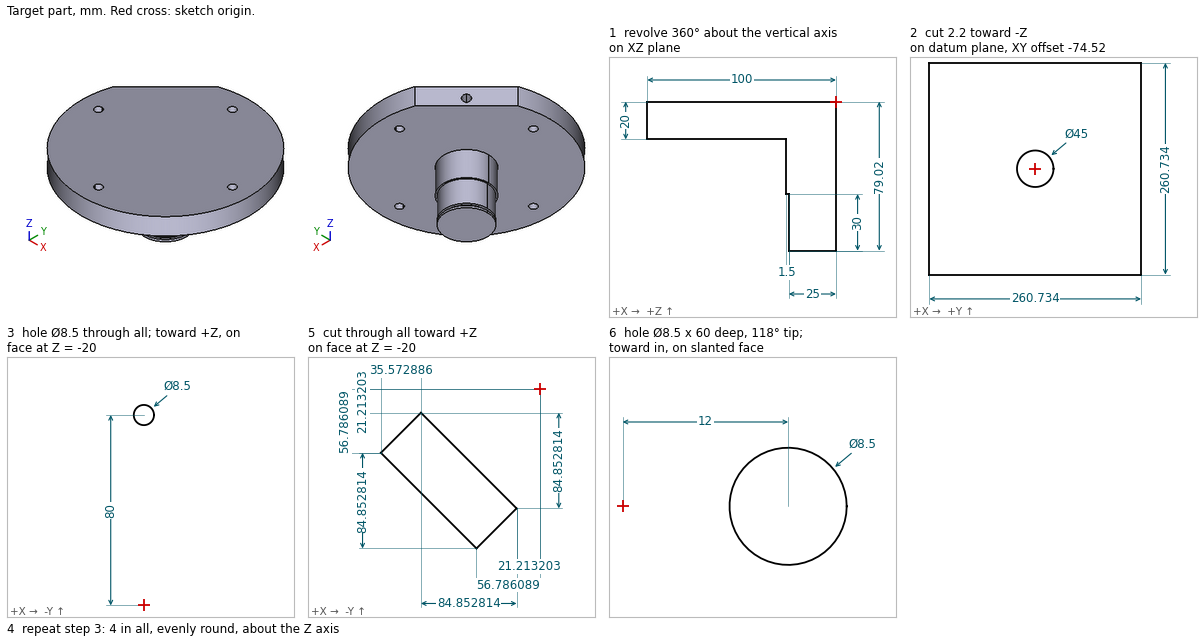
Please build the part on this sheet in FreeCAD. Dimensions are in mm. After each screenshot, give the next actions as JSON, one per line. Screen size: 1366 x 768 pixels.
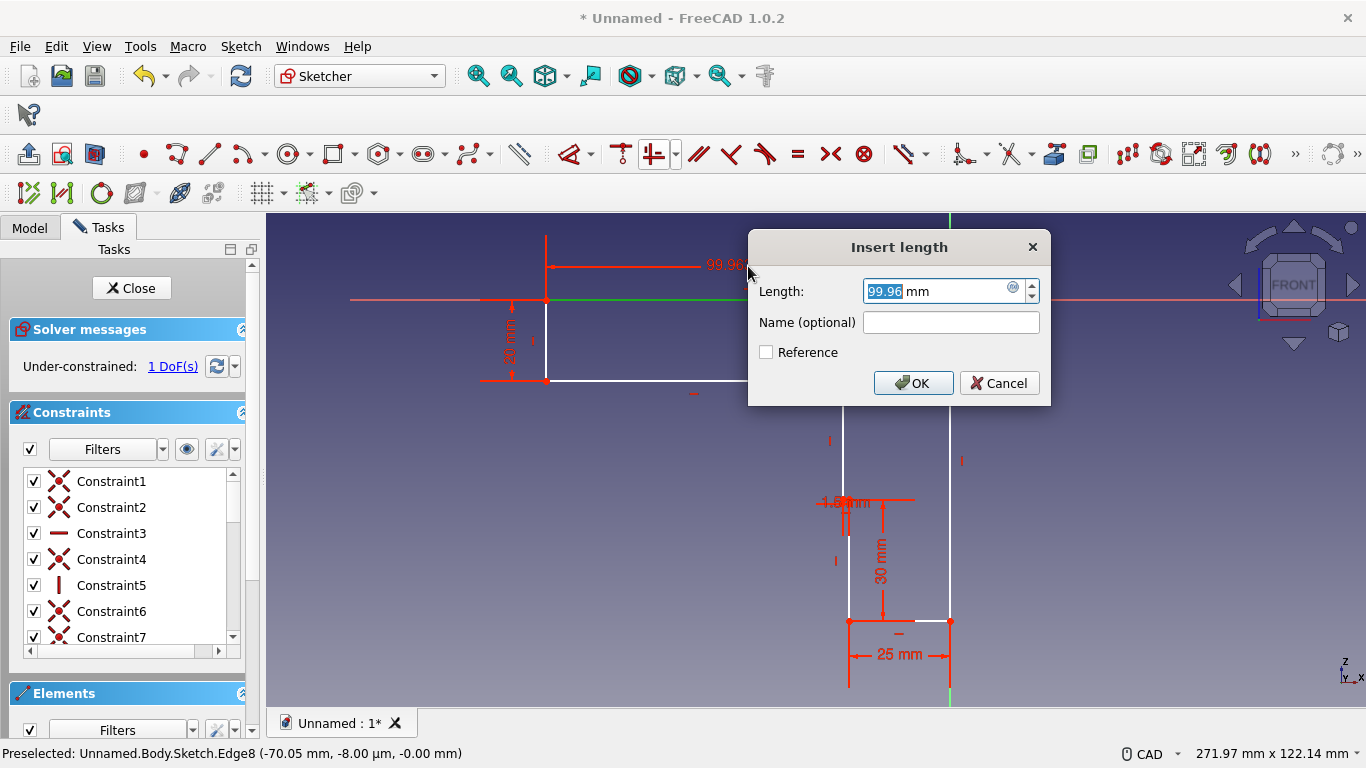
{"action": "type", "text": "100"}
{"action": "key", "text": "Return"}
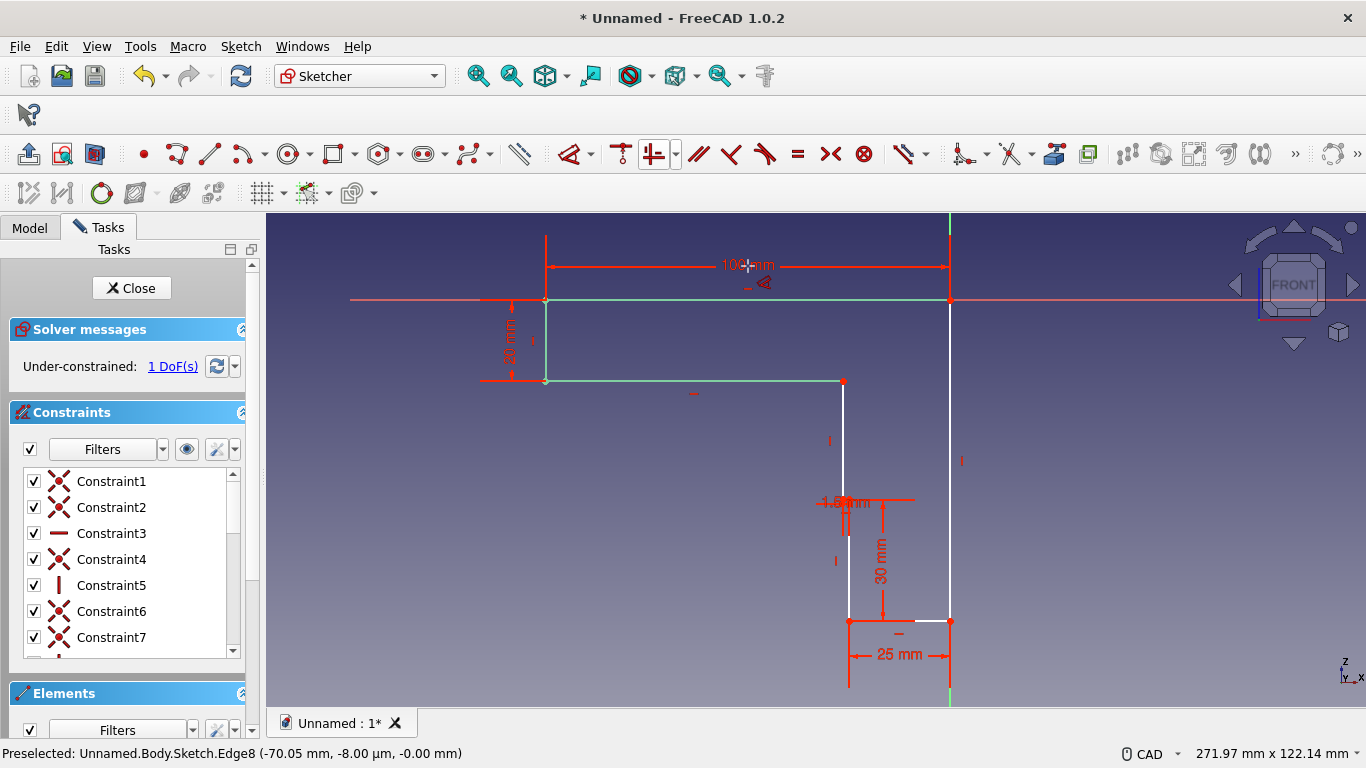
{"action": "left_click", "coordinate": [950, 397]}
{"action": "left_click", "coordinate": [984, 461]}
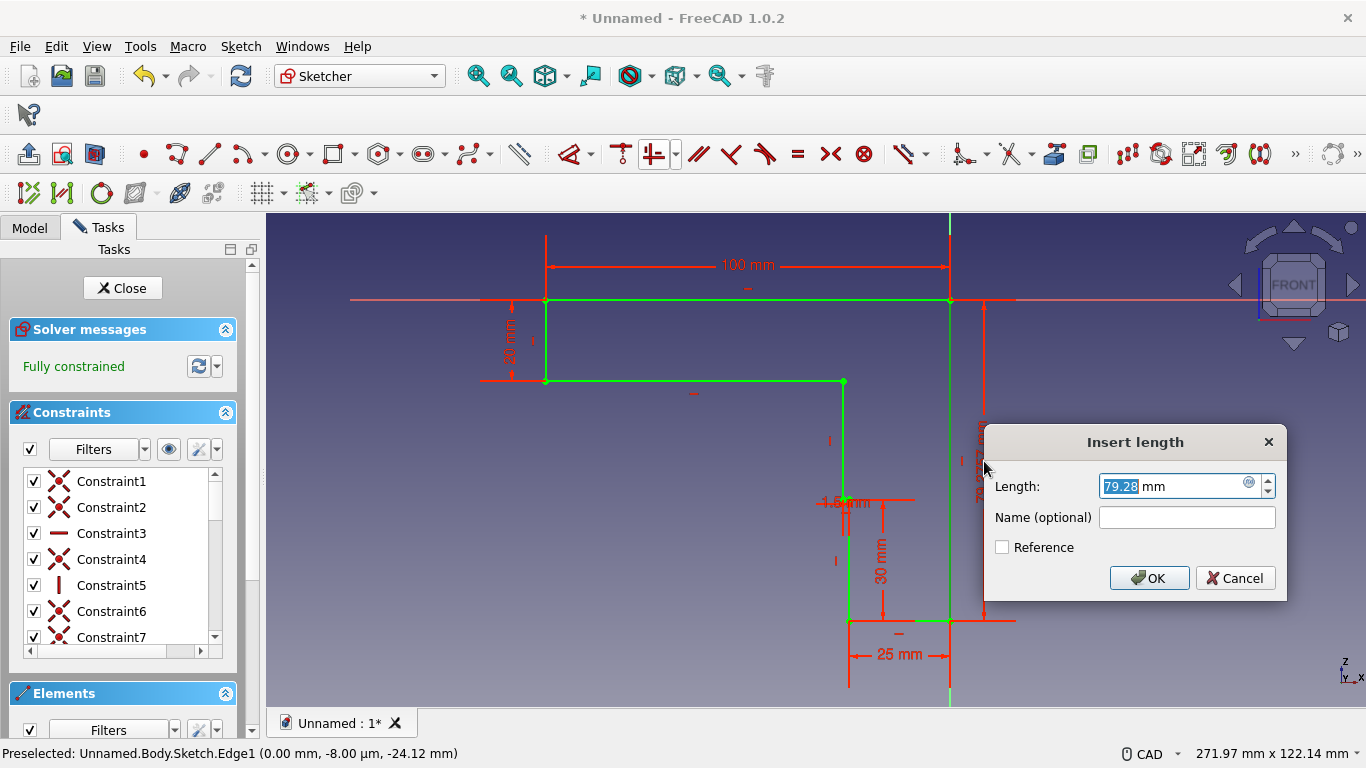
{"action": "type", "text": "79.02"}
{"action": "key", "text": "Return"}
{"action": "key", "text": "Escape"}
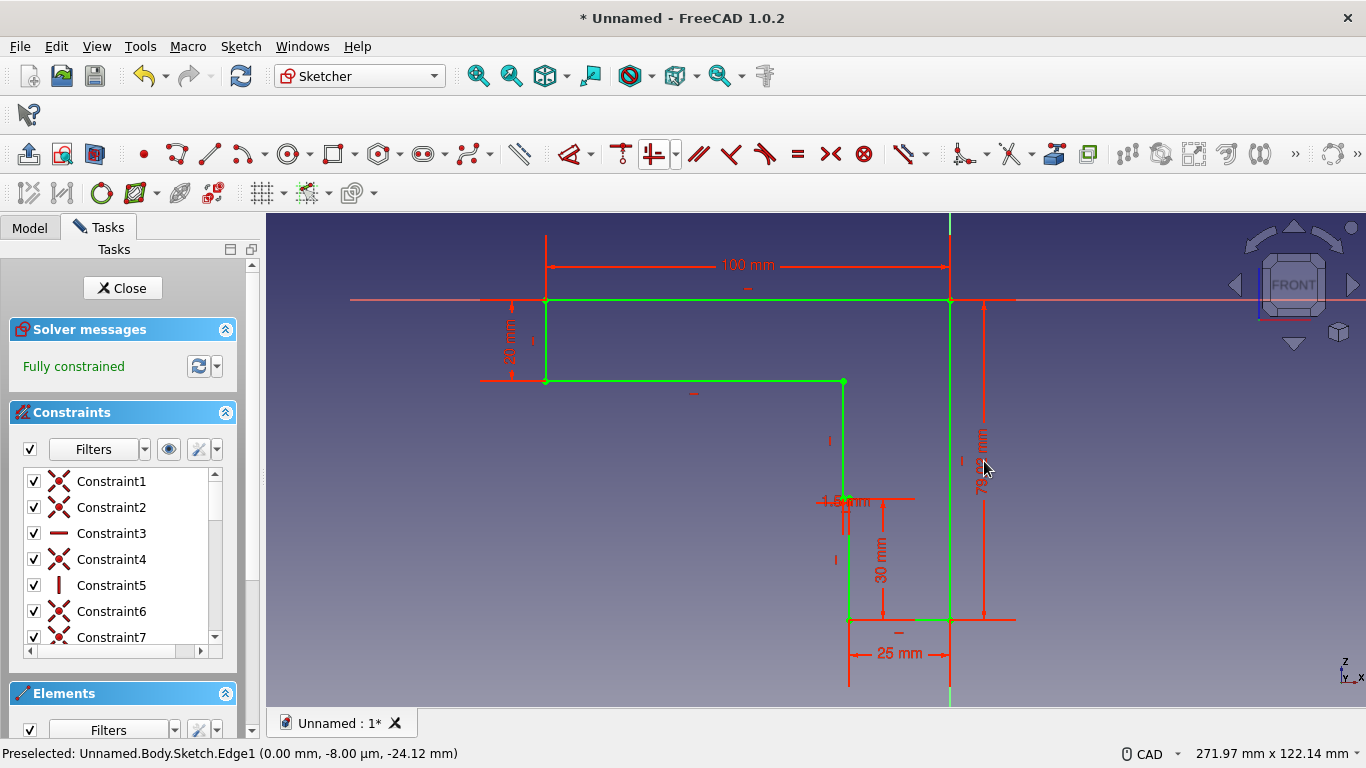
{"action": "left_click", "coordinate": [123, 288]}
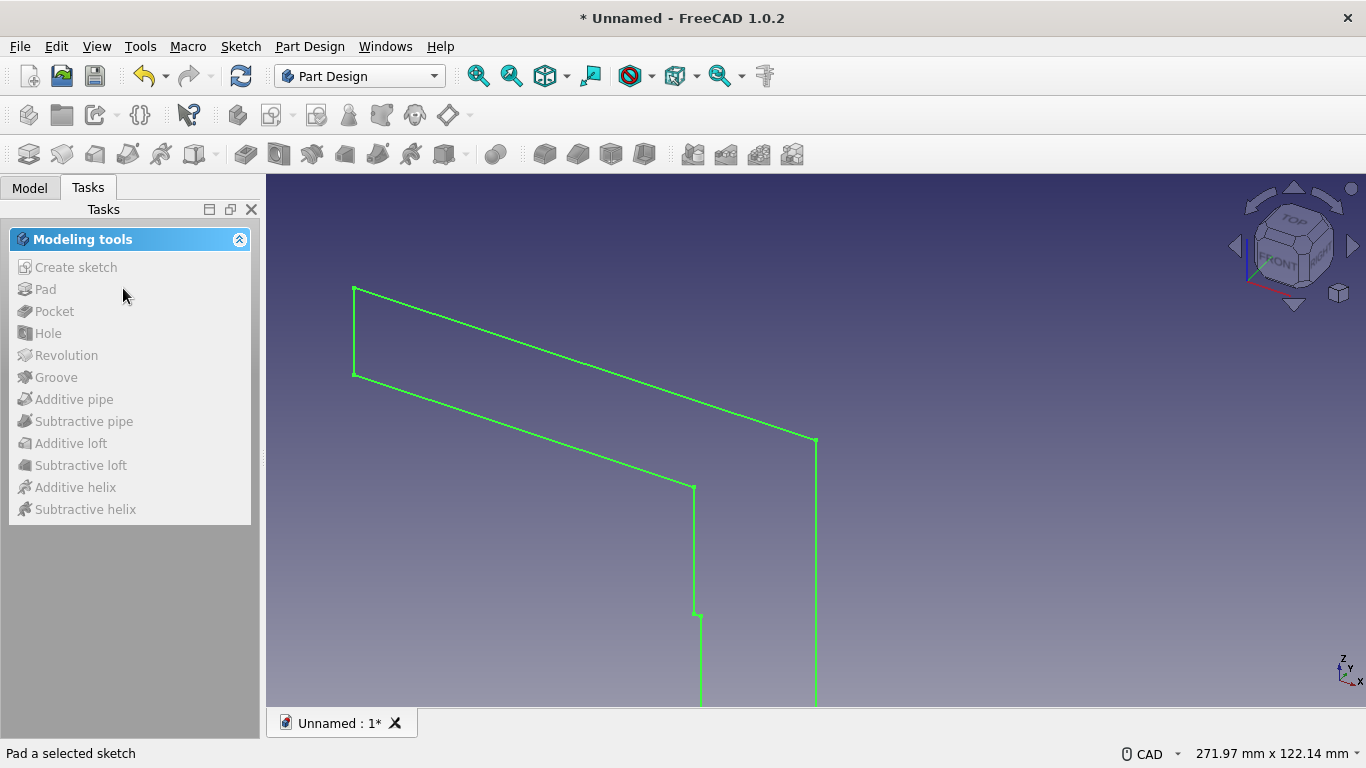
{"action": "left_click", "coordinate": [62, 154]}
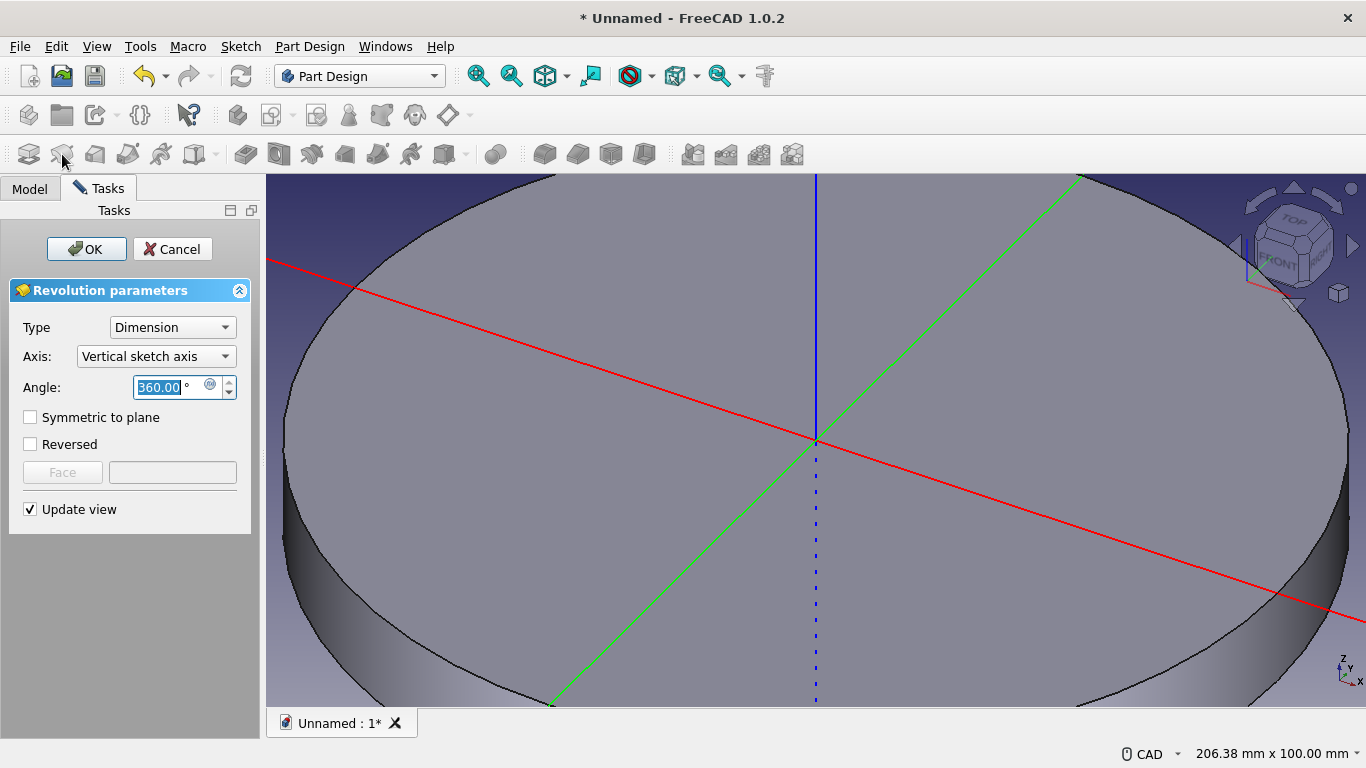
{"action": "left_click", "coordinate": [87, 249]}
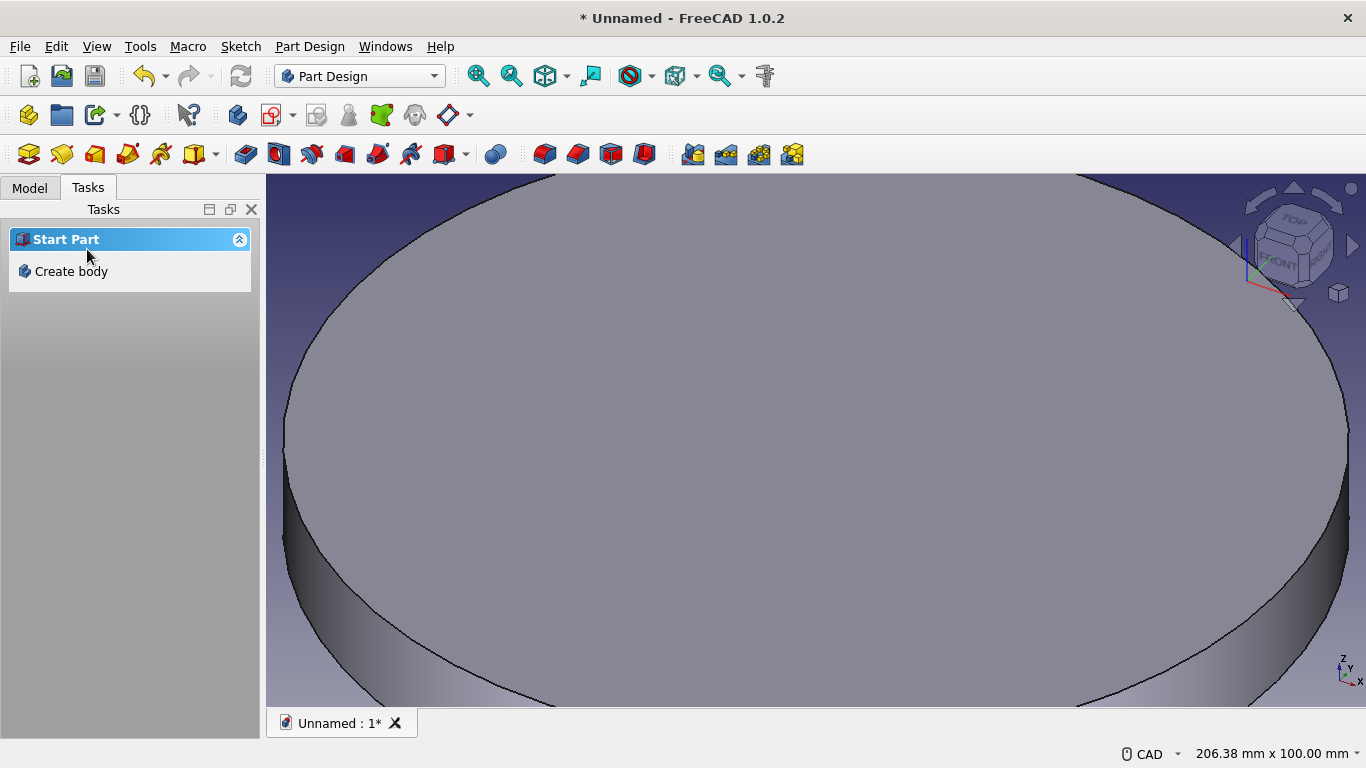
{"action": "left_click", "coordinate": [479, 76]}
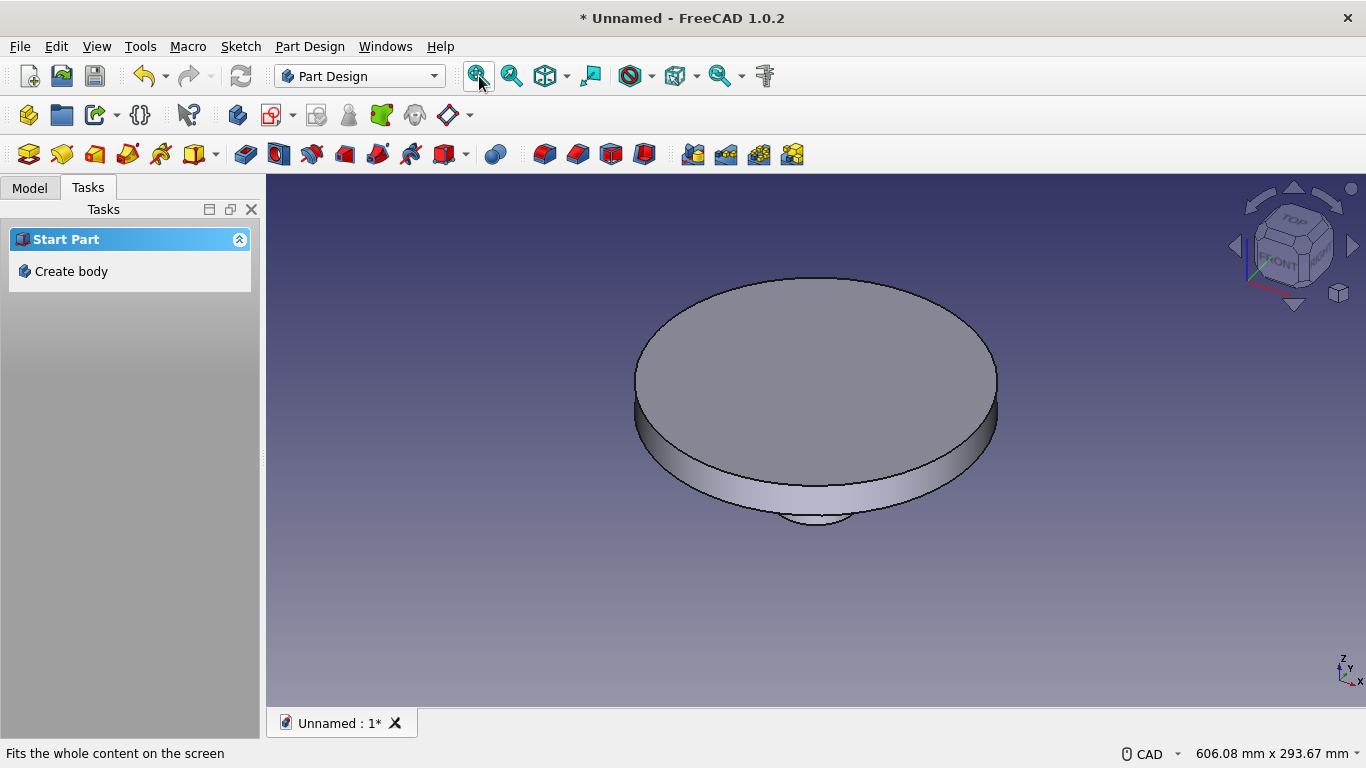
{"action": "left_click", "coordinate": [30, 188]}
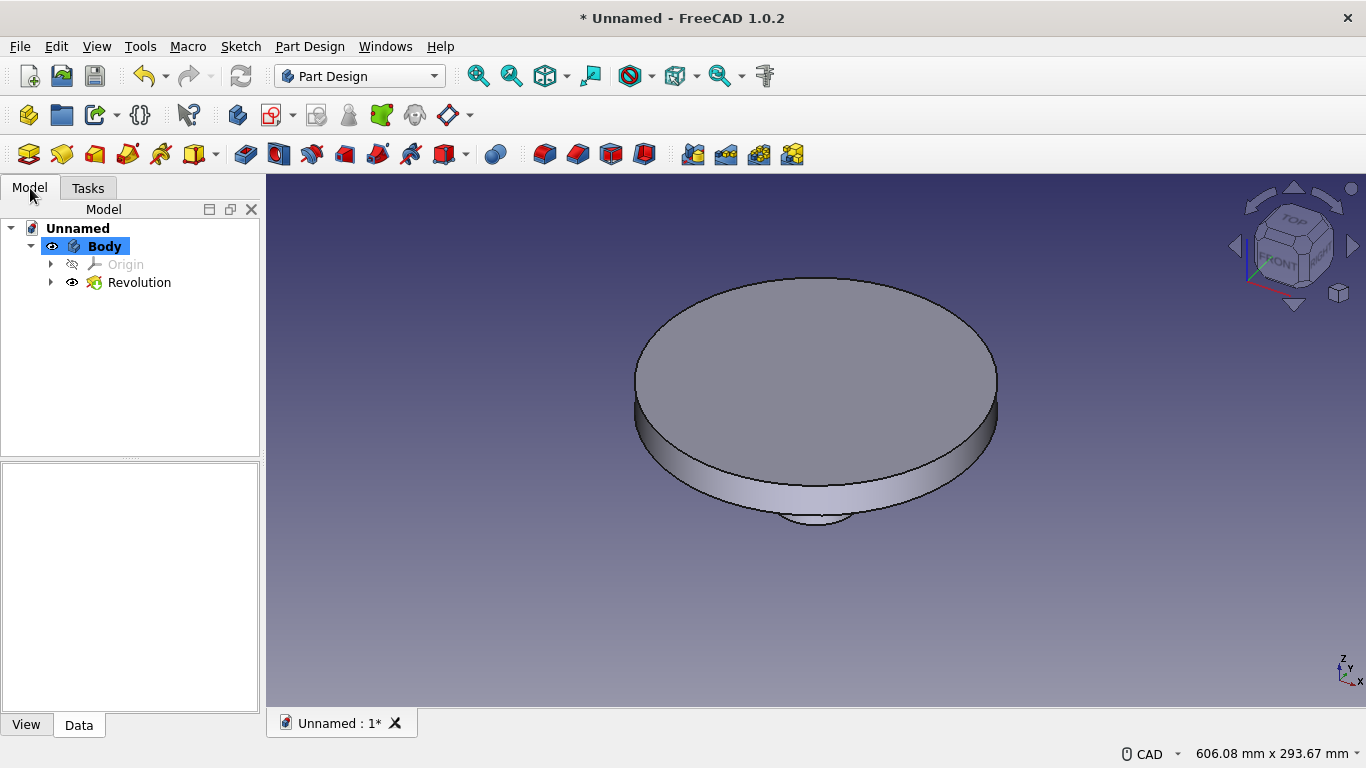
{"action": "left_click", "coordinate": [51, 264]}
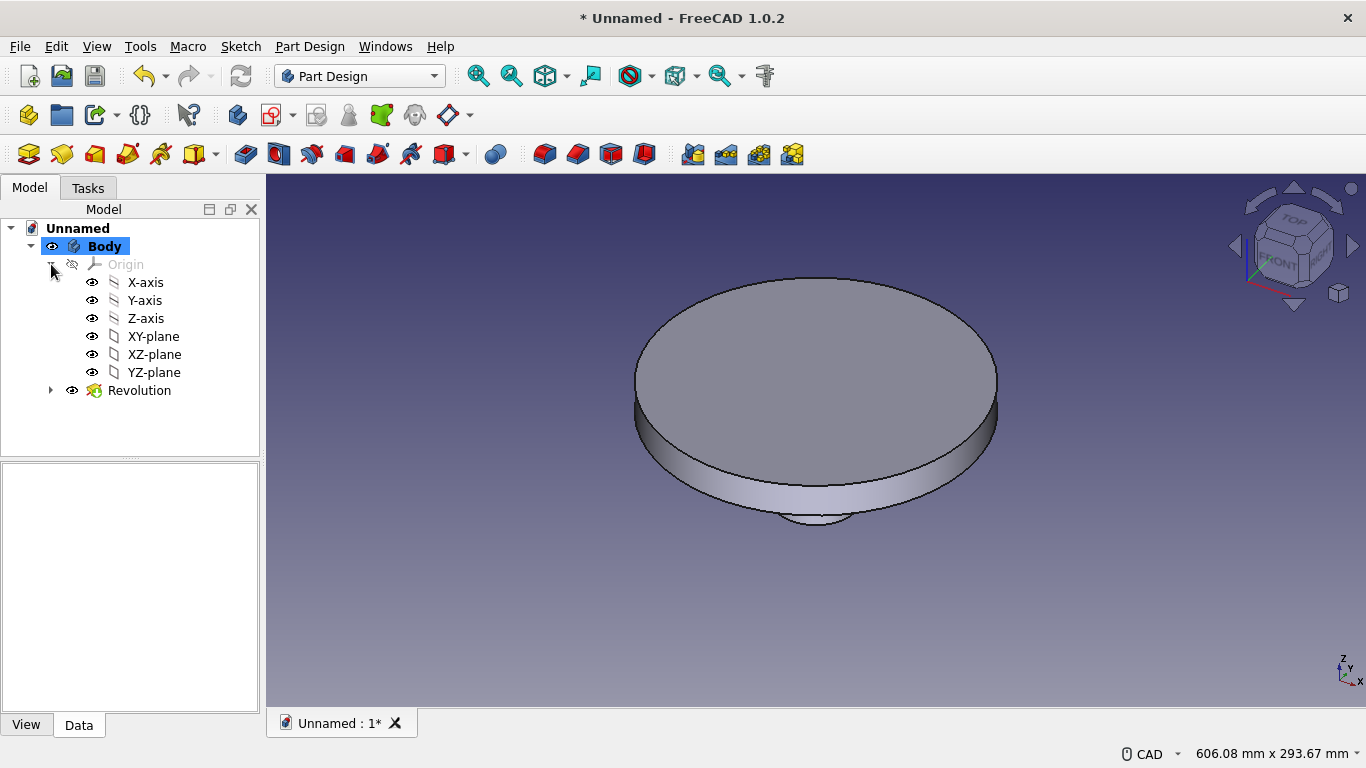
{"action": "left_click", "coordinate": [137, 336]}